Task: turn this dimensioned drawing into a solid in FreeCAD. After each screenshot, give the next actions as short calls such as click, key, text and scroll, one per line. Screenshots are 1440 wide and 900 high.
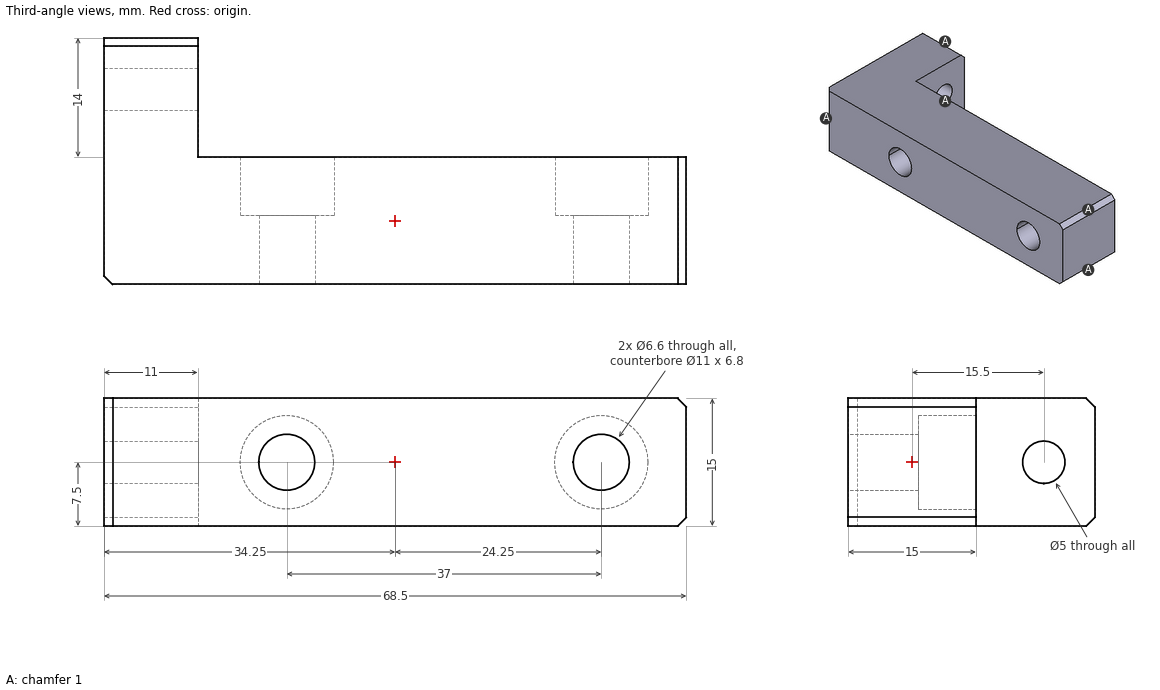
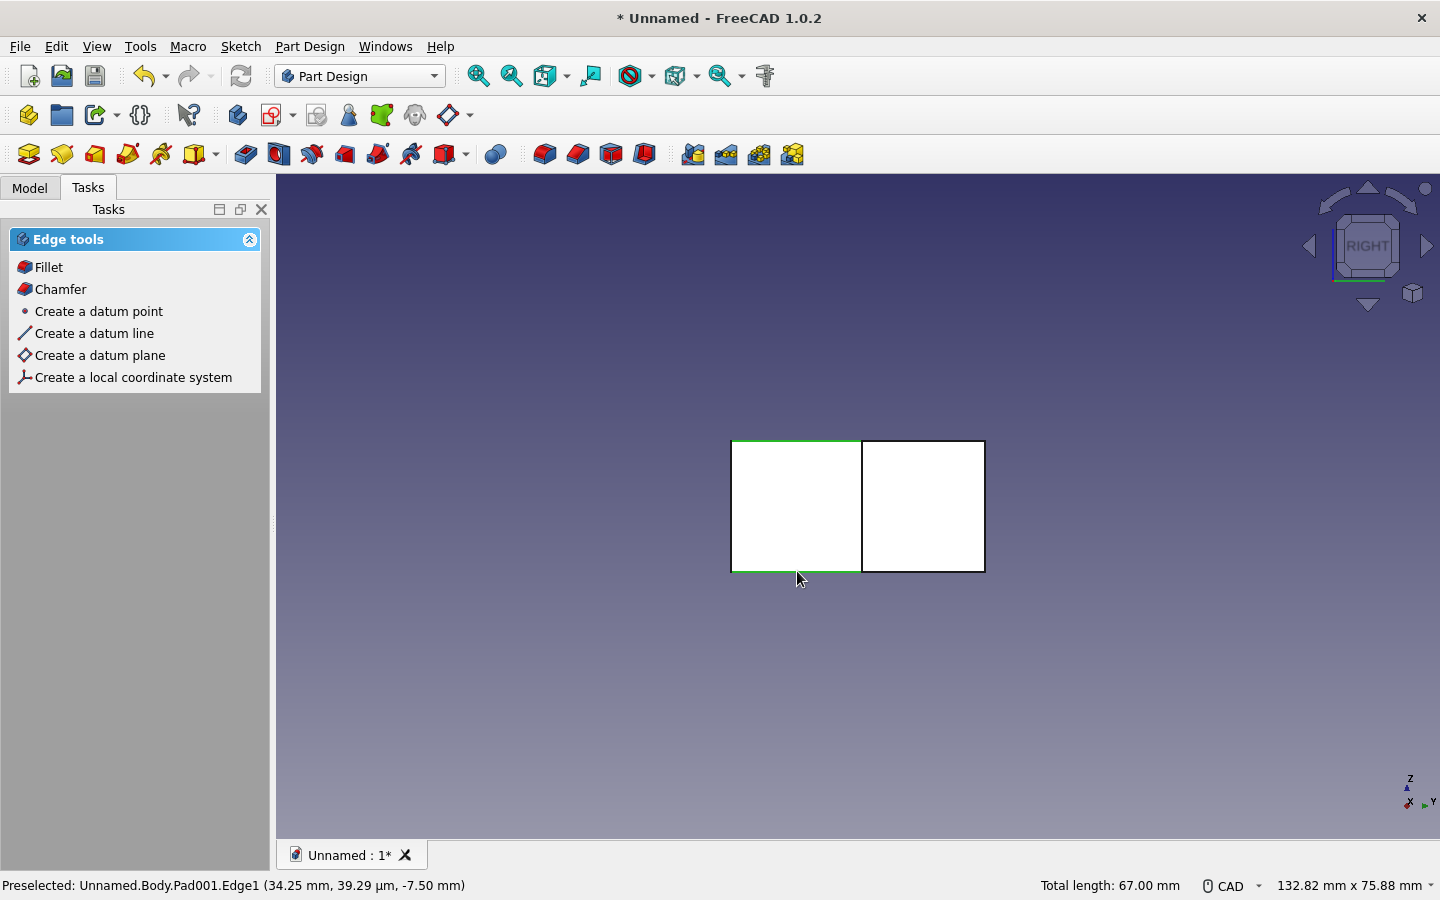
click(578, 154)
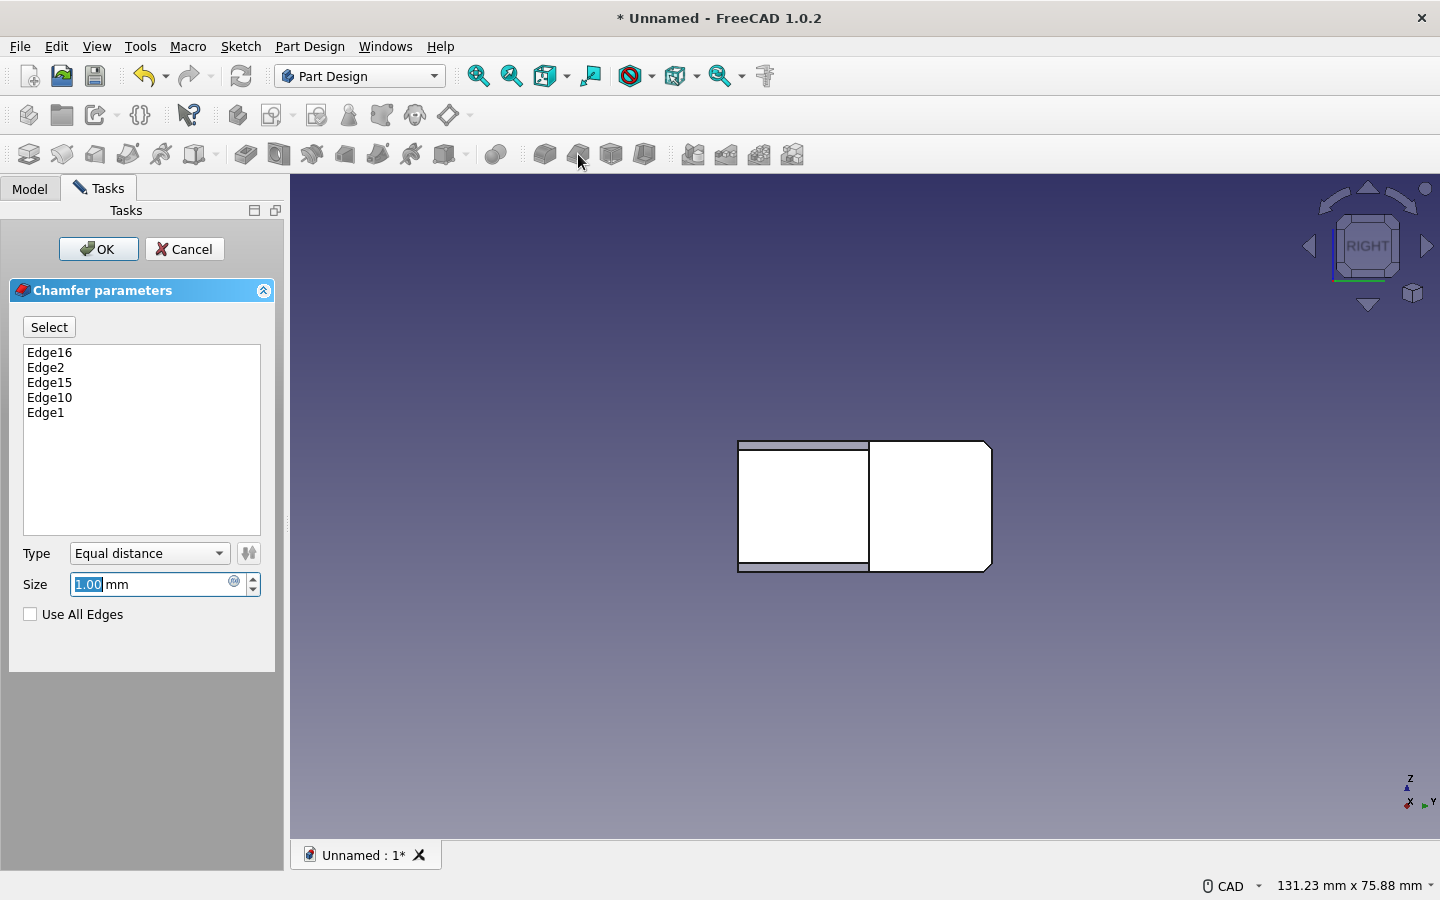
text(1)
key(Tab)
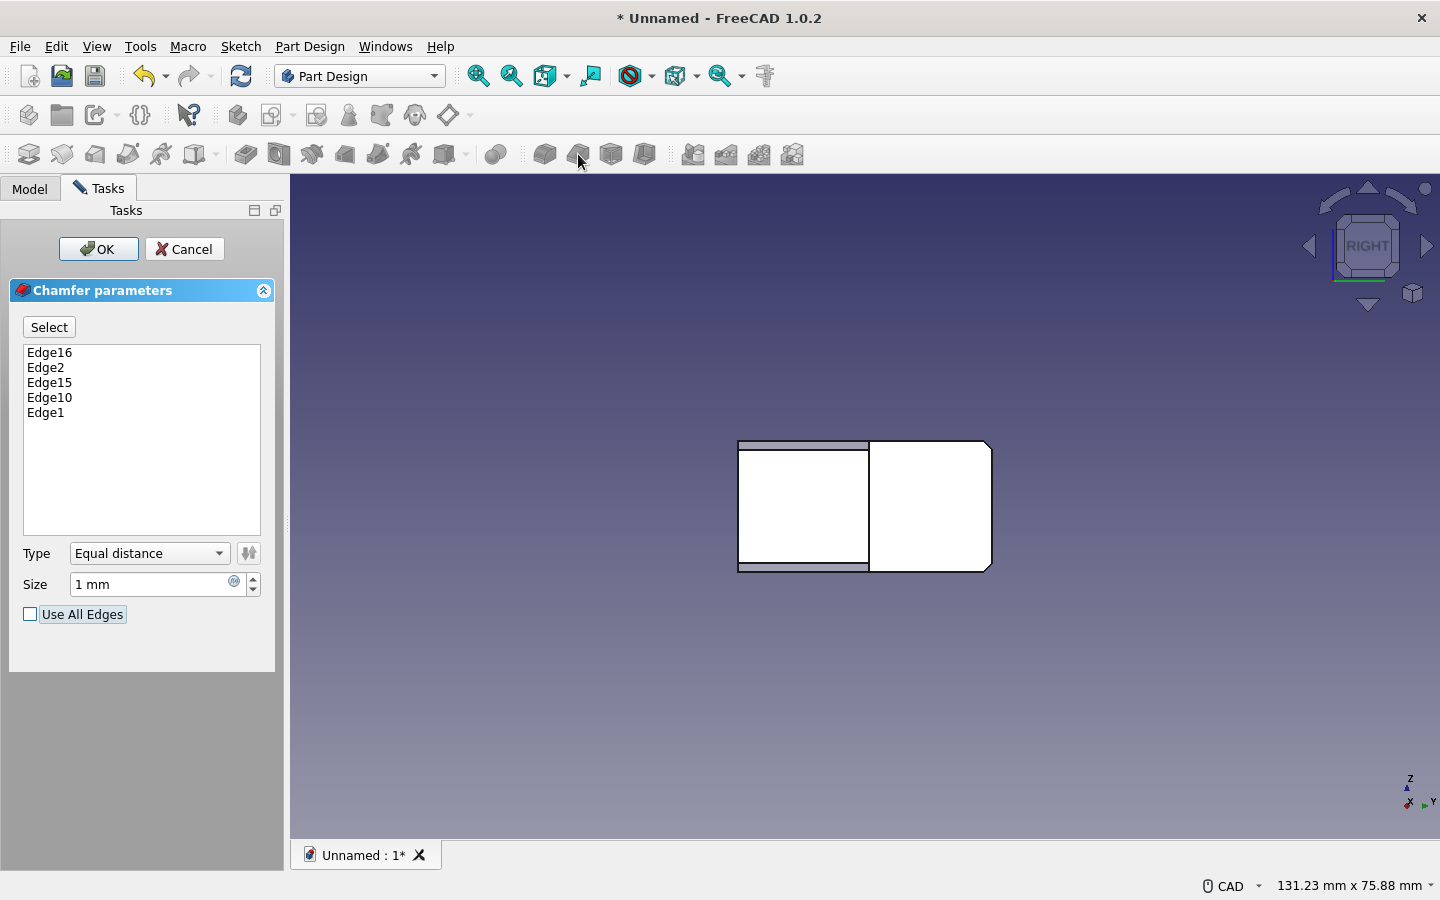
click(99, 249)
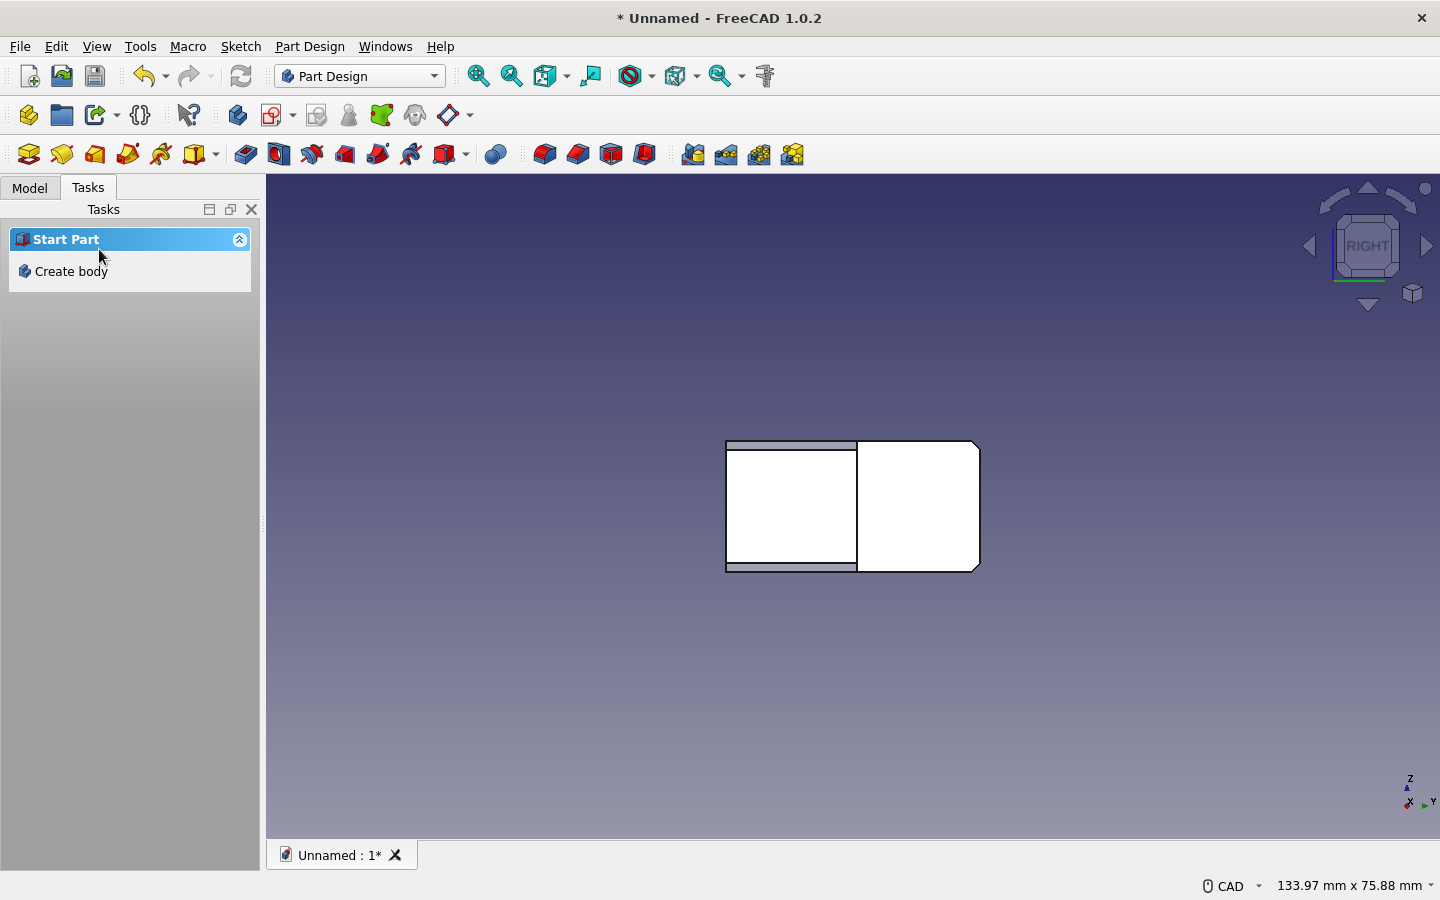
click(479, 76)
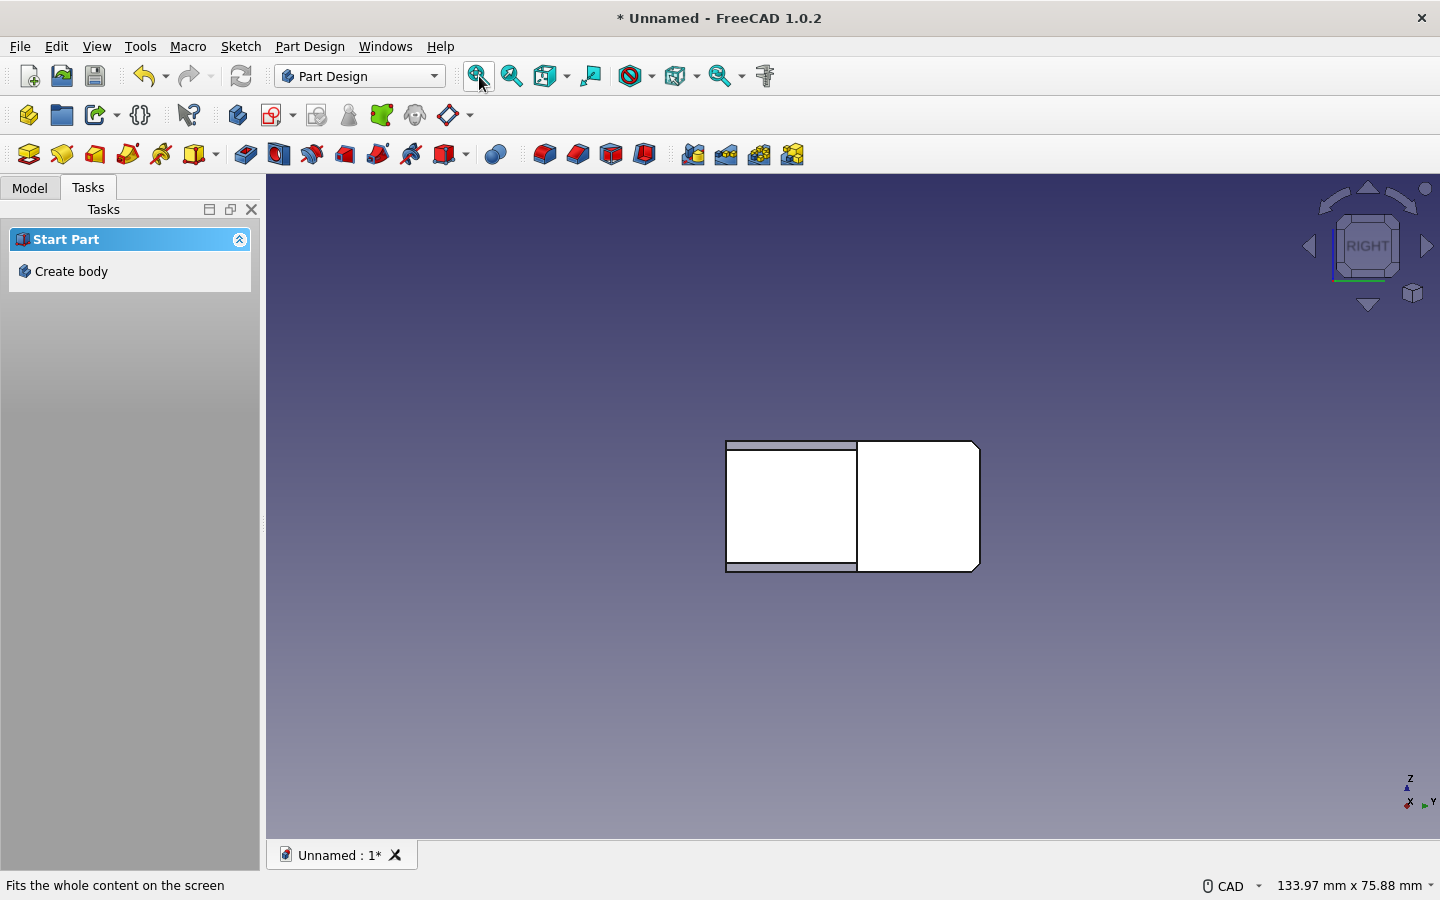
key(4)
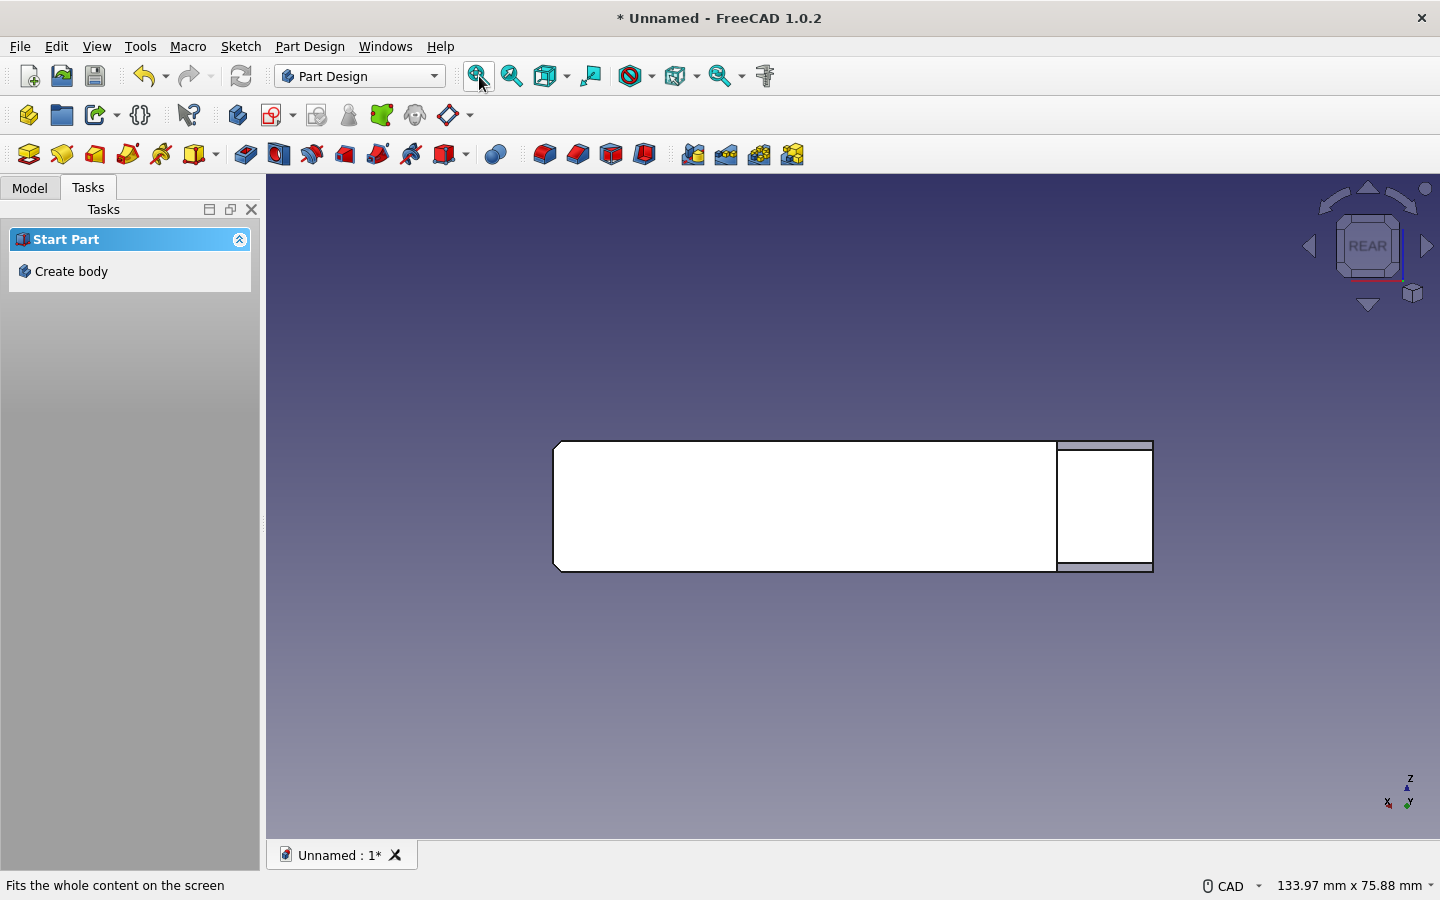
click(661, 505)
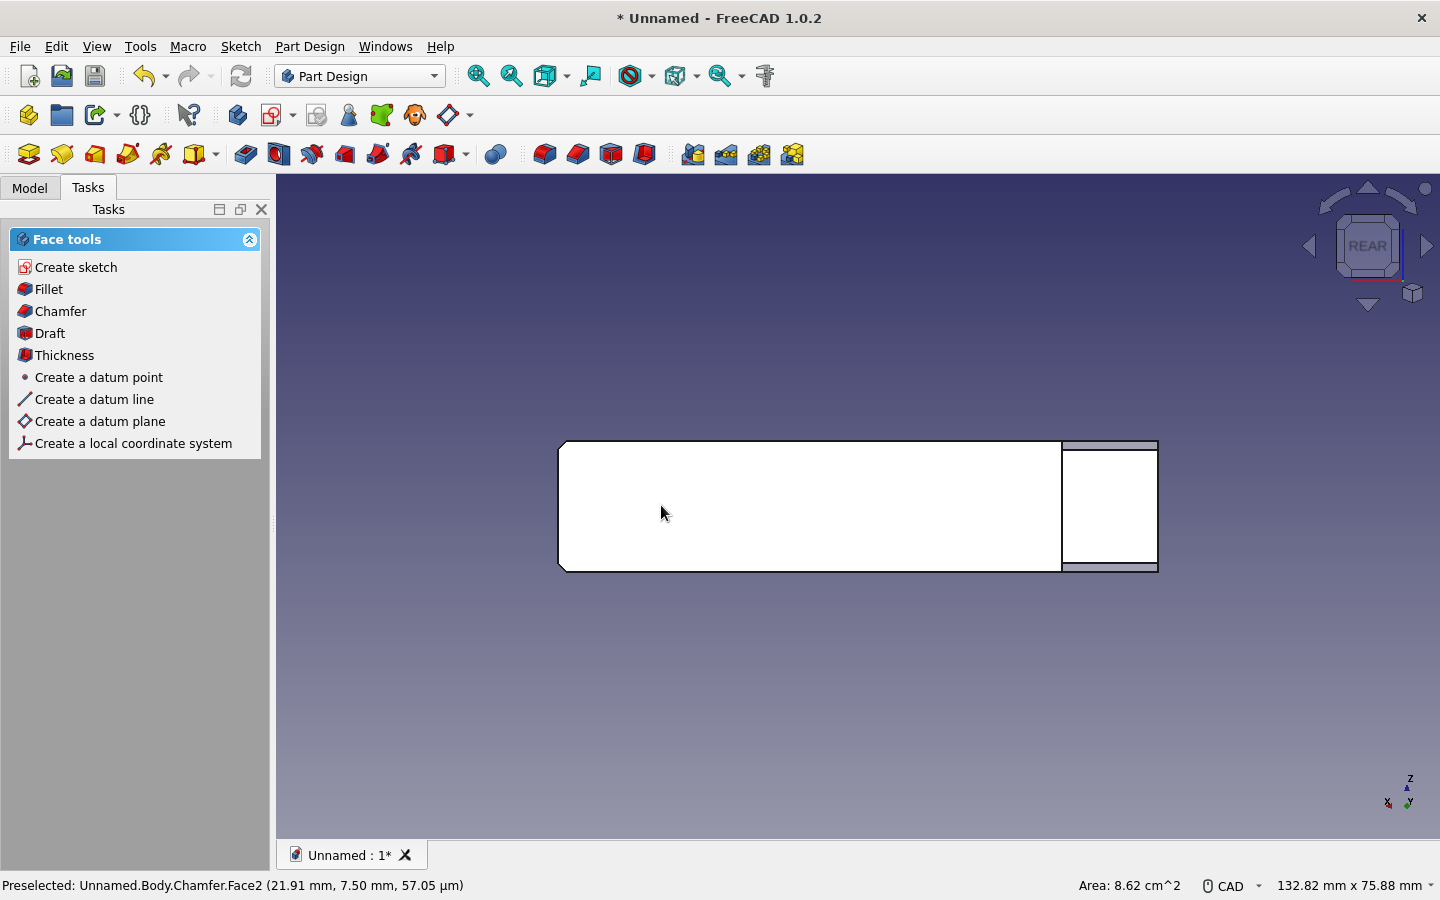
click(270, 116)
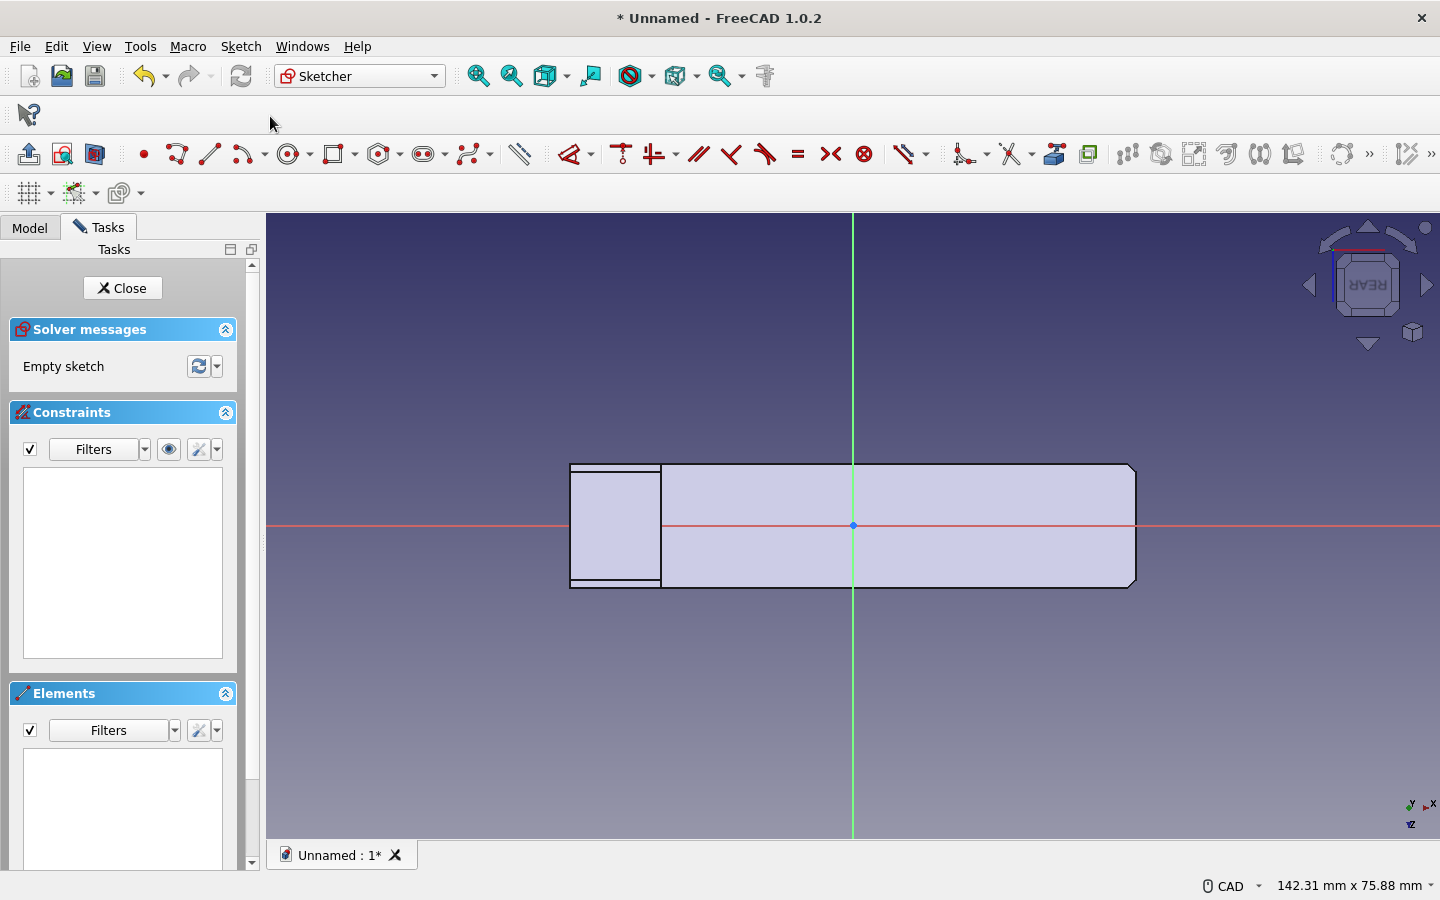
scroll(1041, 526, up, 3)